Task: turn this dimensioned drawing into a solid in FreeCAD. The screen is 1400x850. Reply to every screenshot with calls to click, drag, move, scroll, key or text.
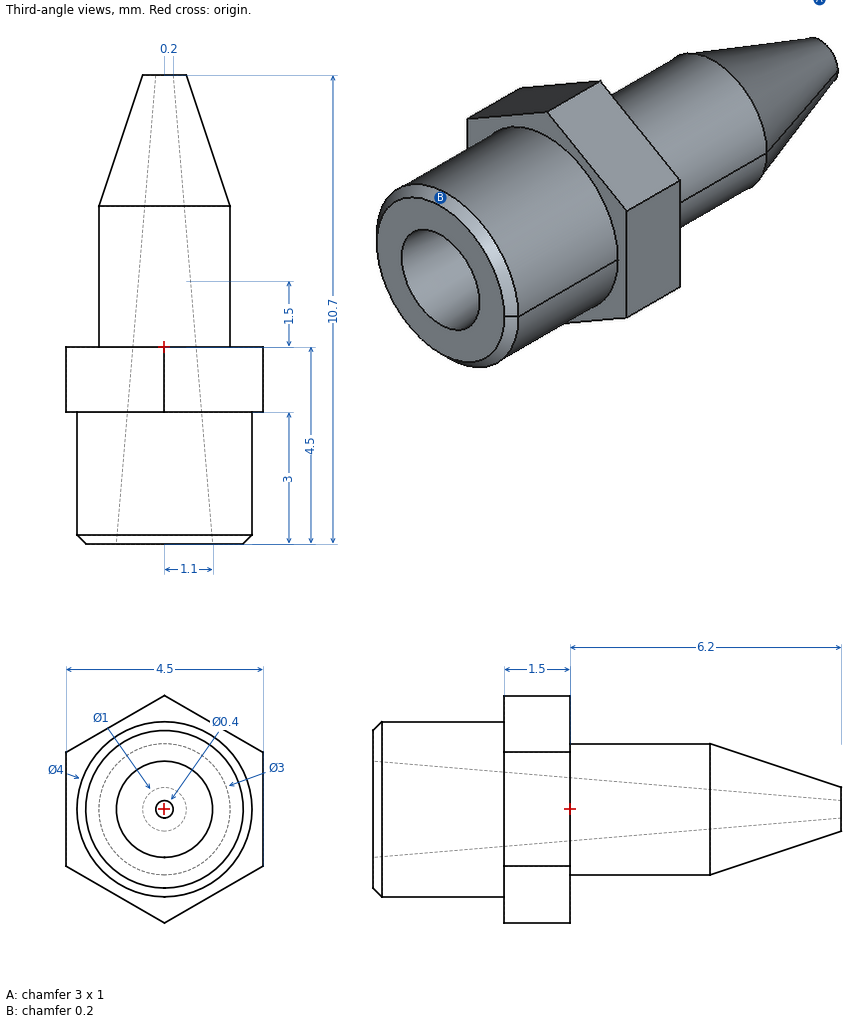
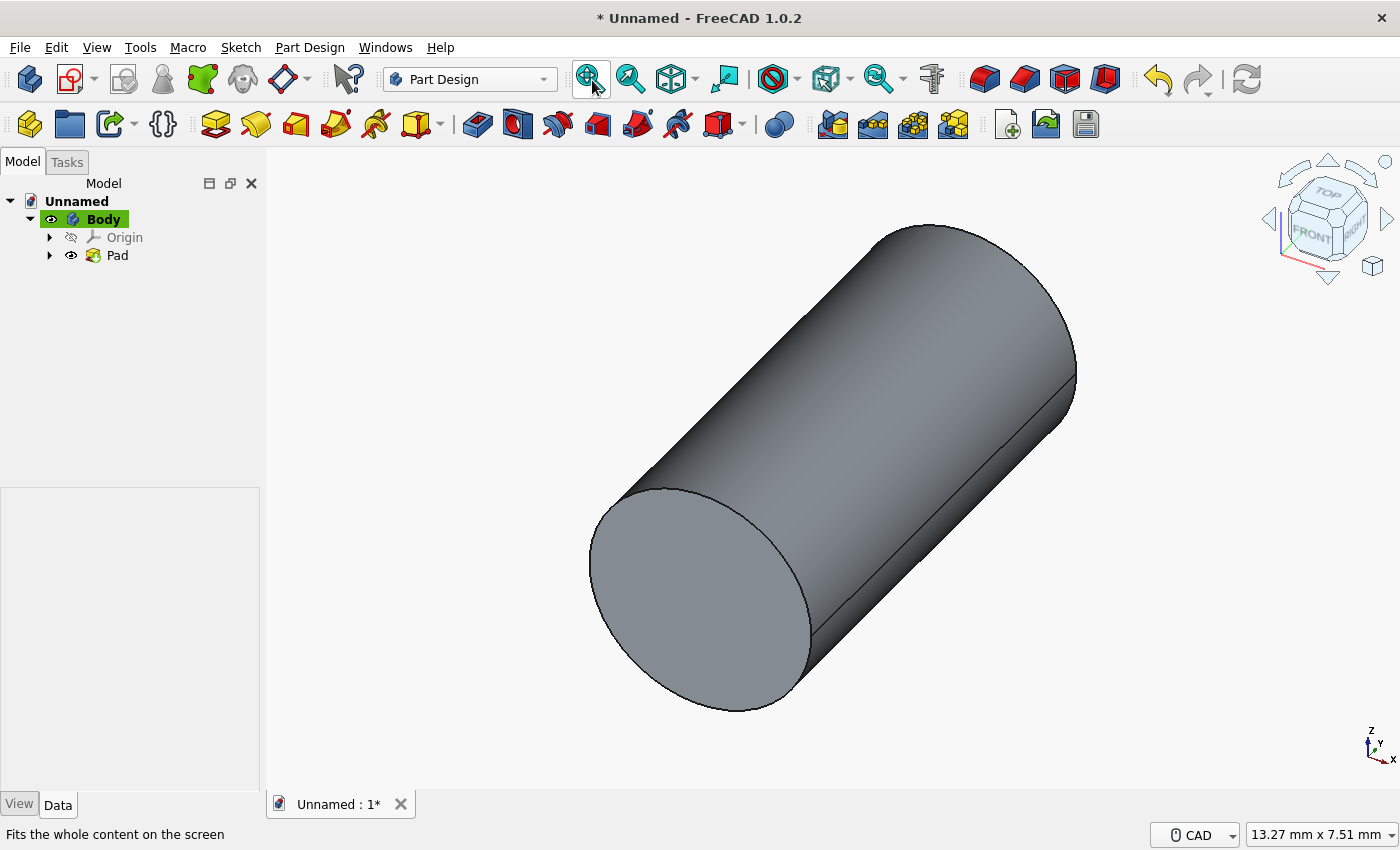
key(4)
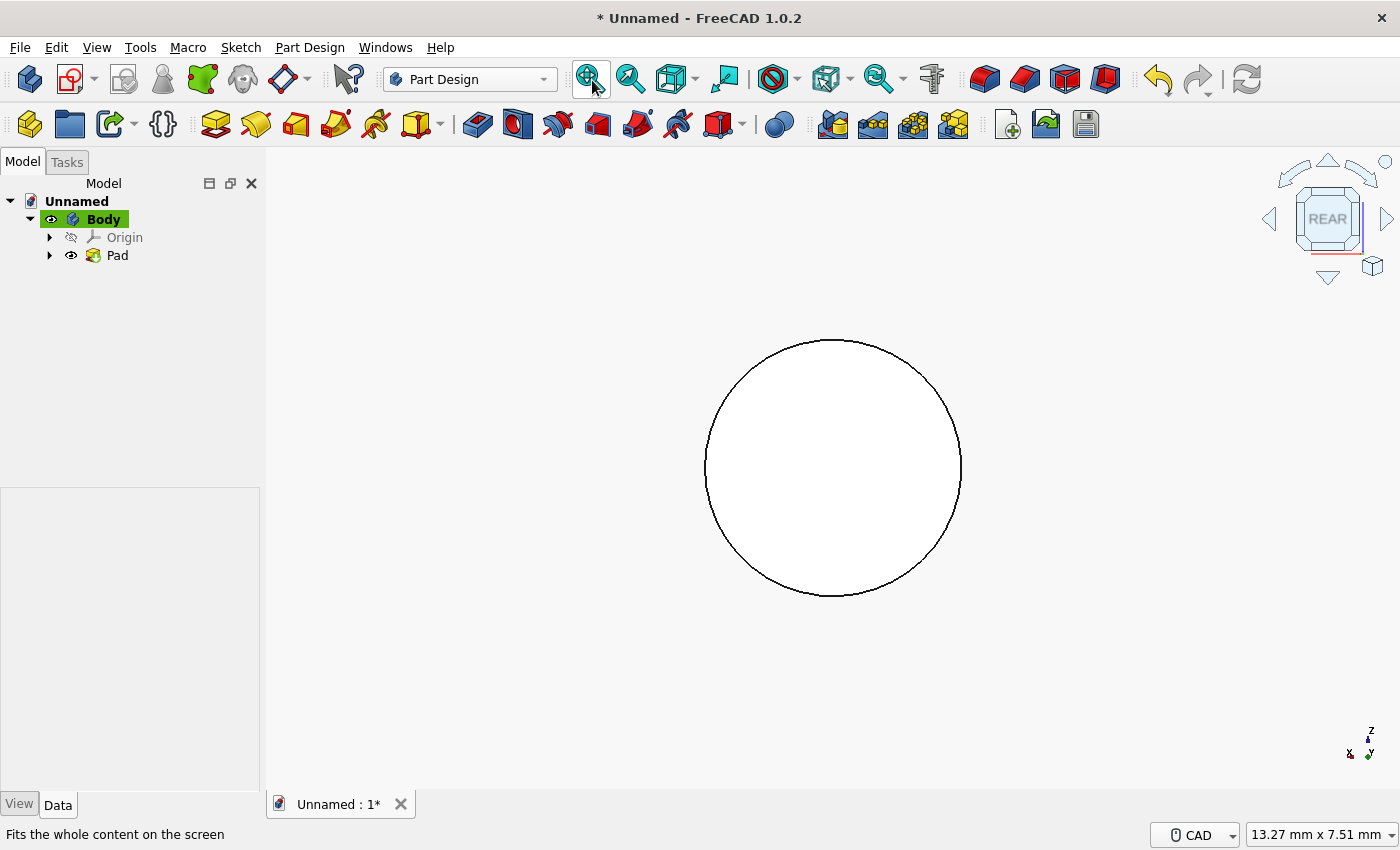
click(592, 80)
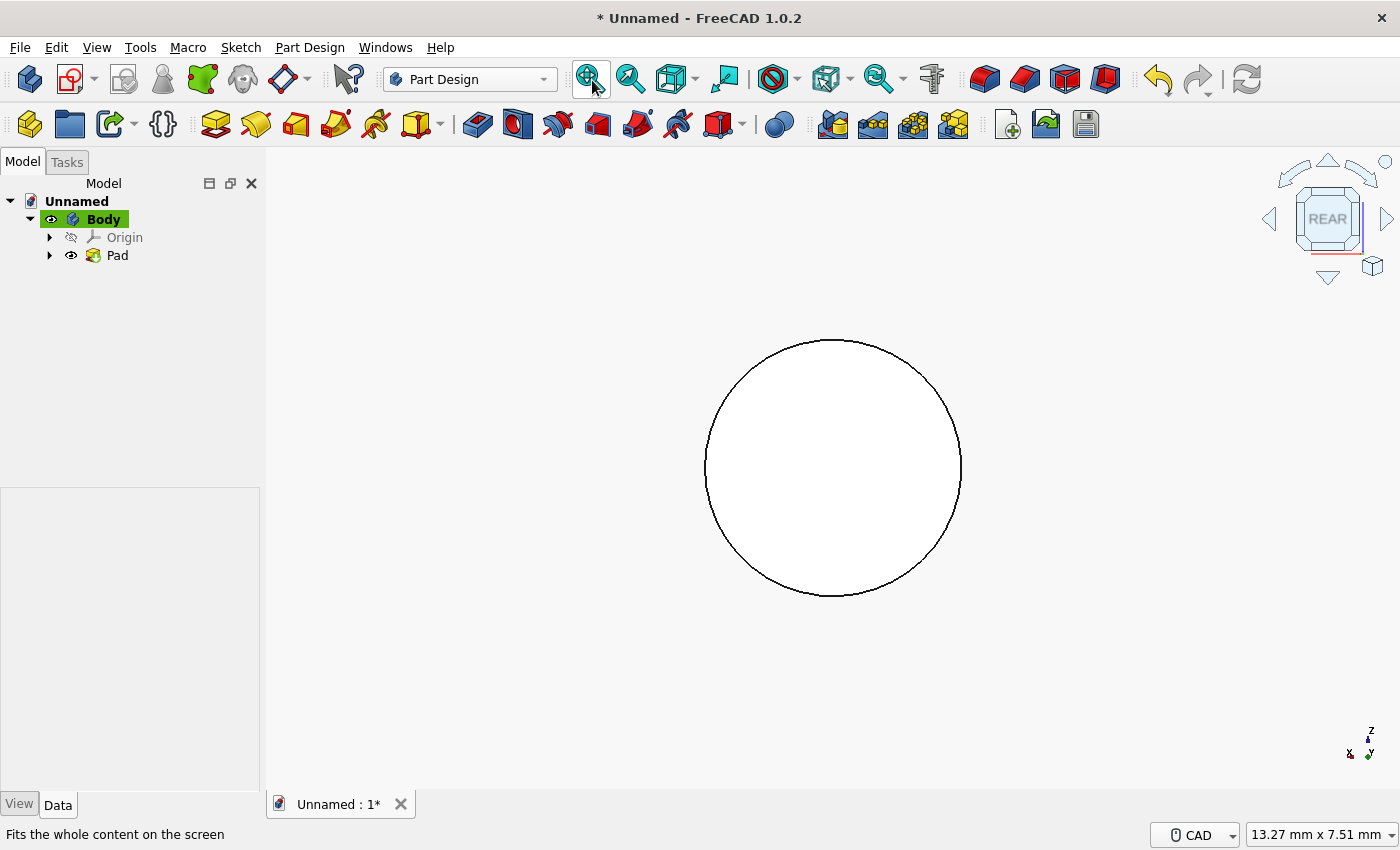
click(833, 467)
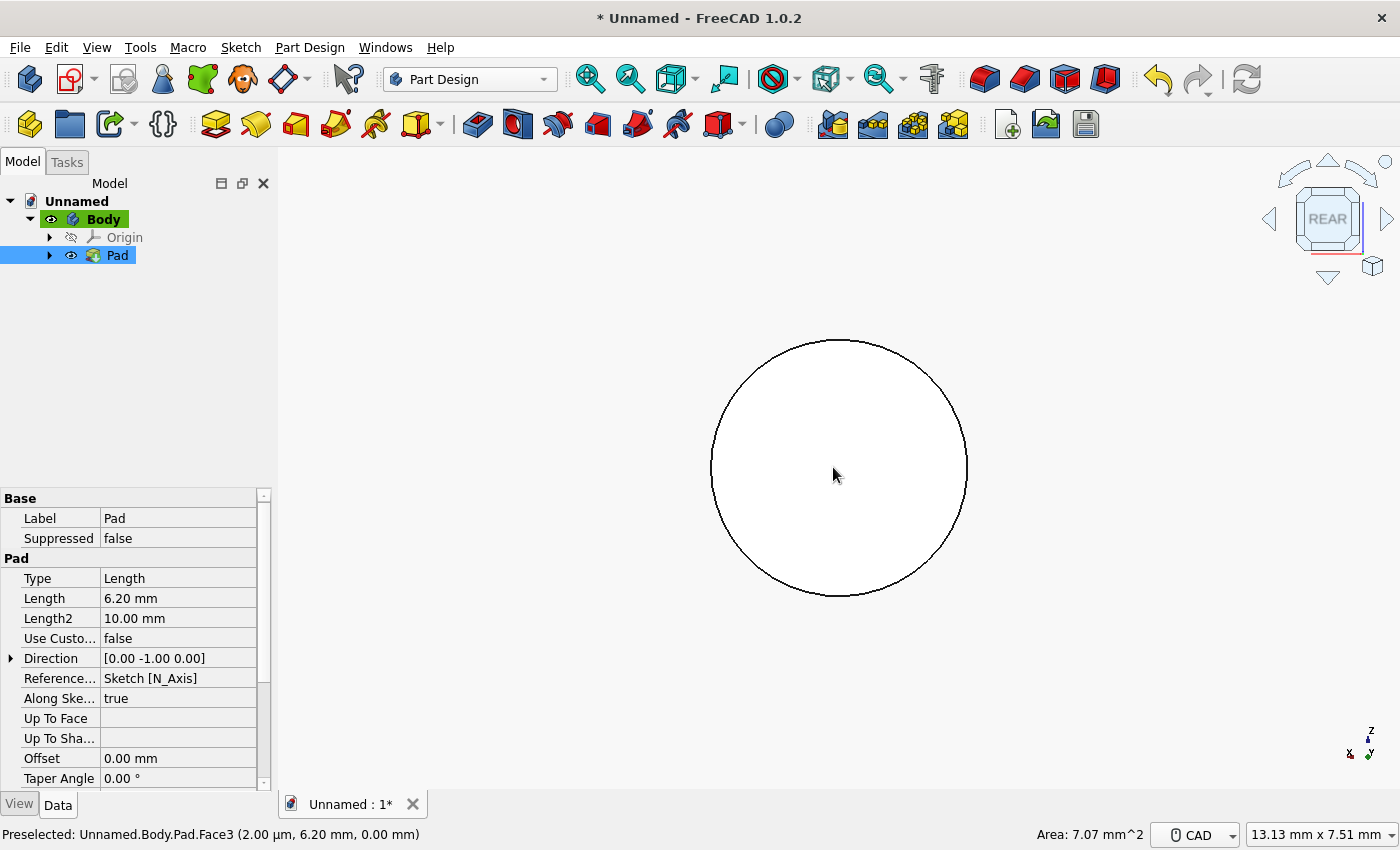
click(70, 80)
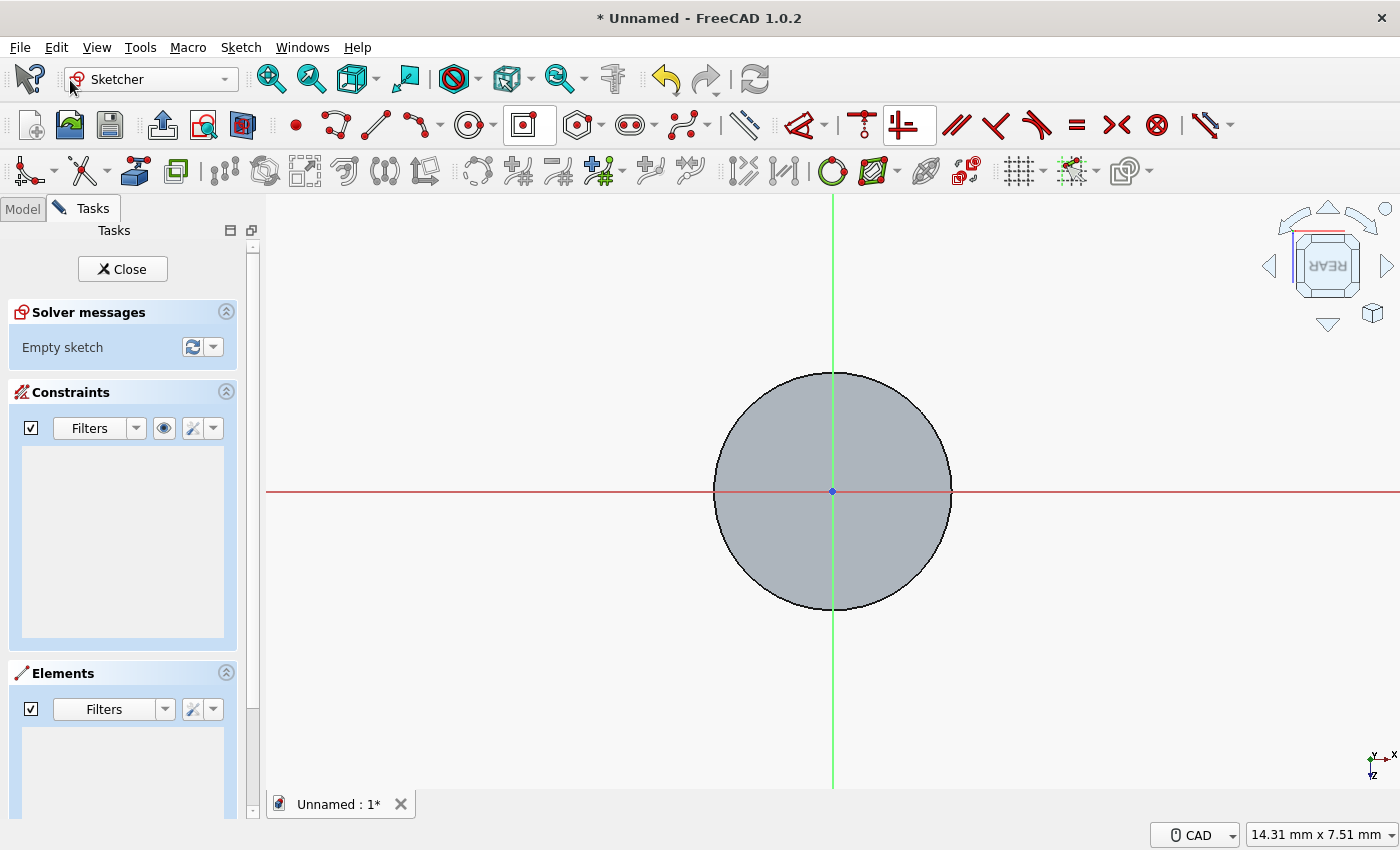
scroll(840, 491, up, 12)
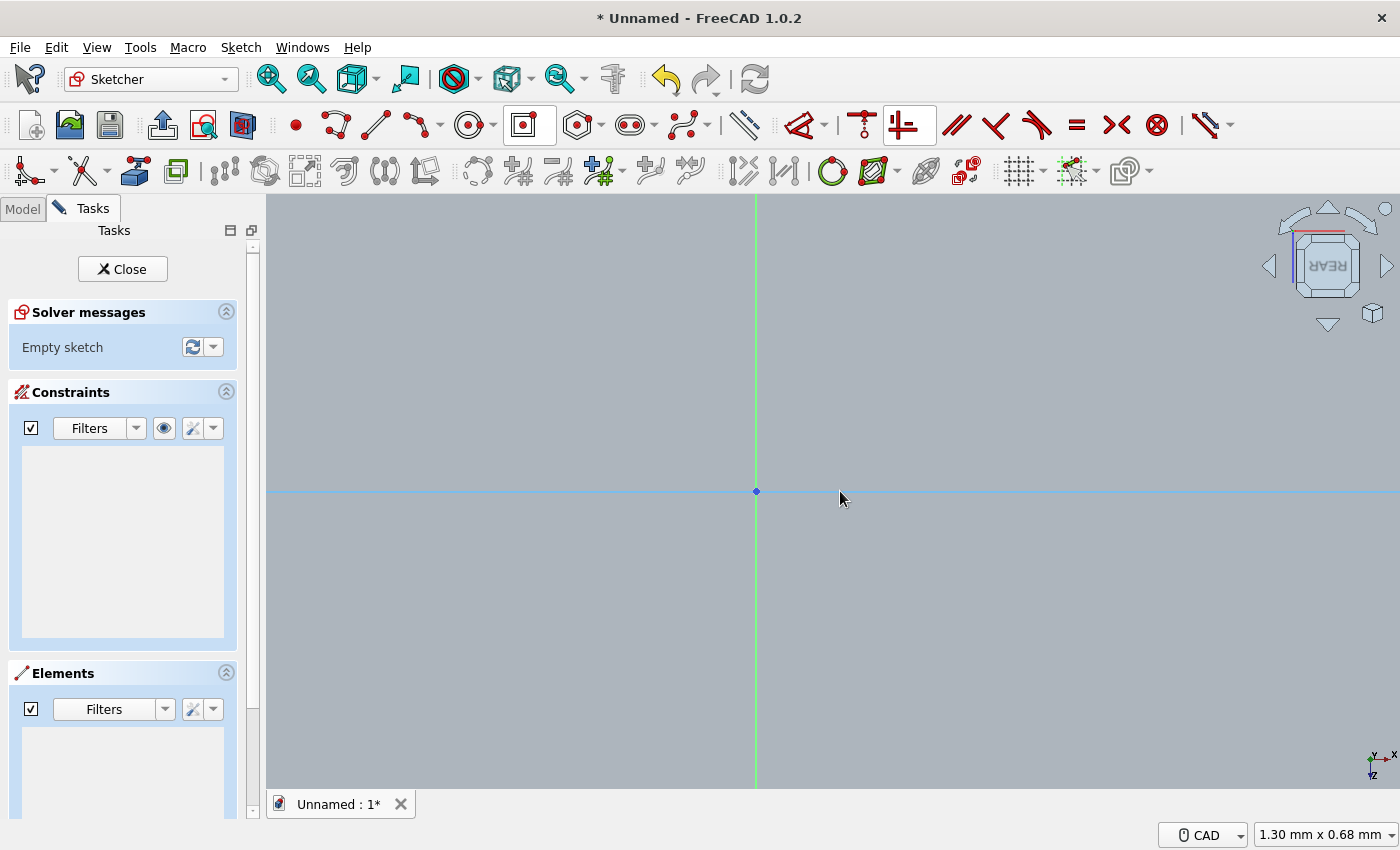
click(470, 126)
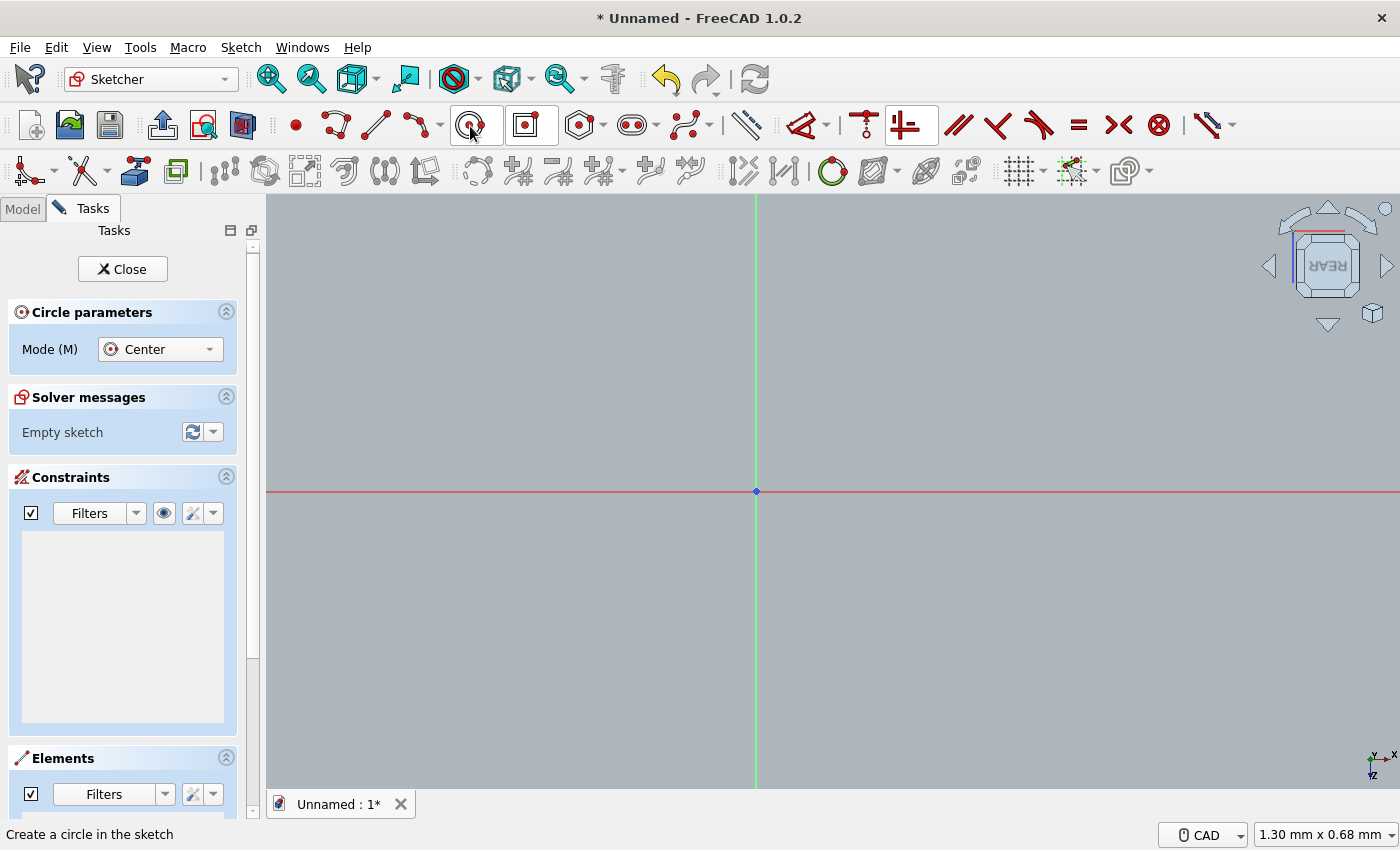
click(756, 491)
click(880, 368)
key(Escape)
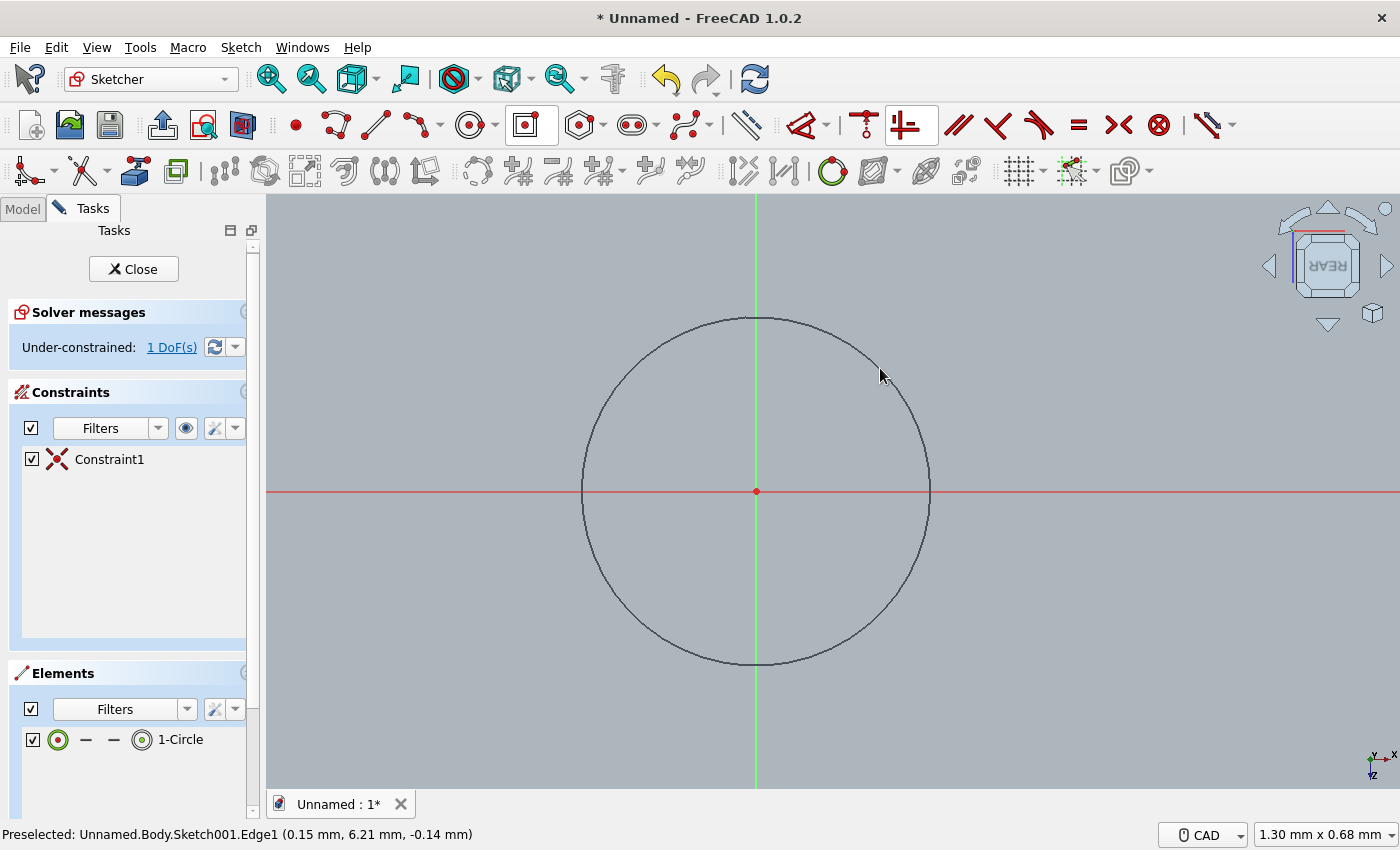
click(879, 368)